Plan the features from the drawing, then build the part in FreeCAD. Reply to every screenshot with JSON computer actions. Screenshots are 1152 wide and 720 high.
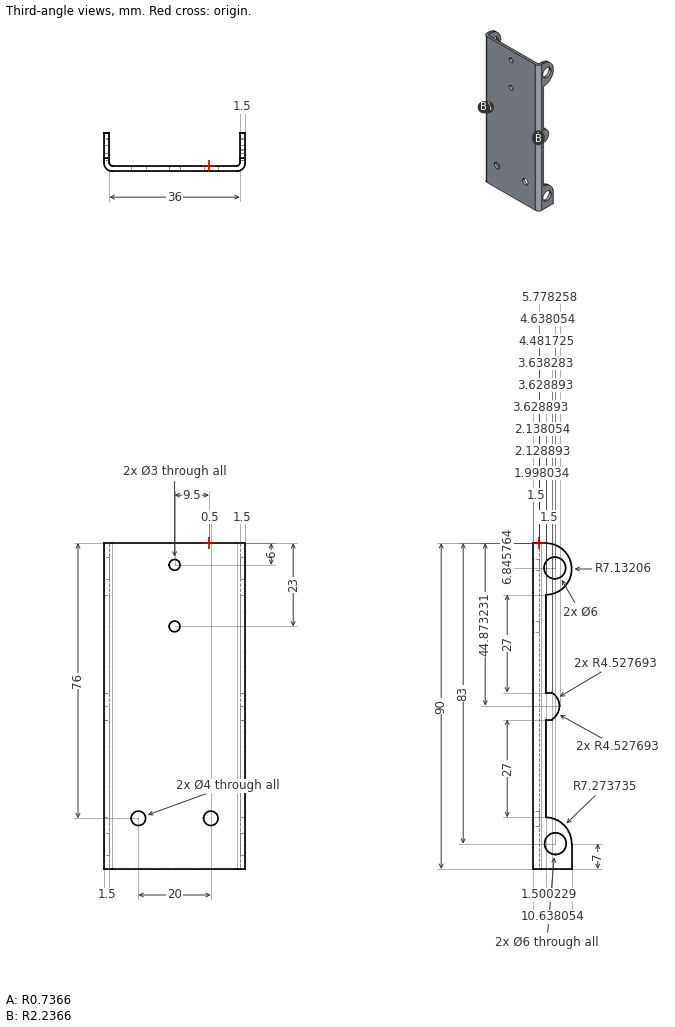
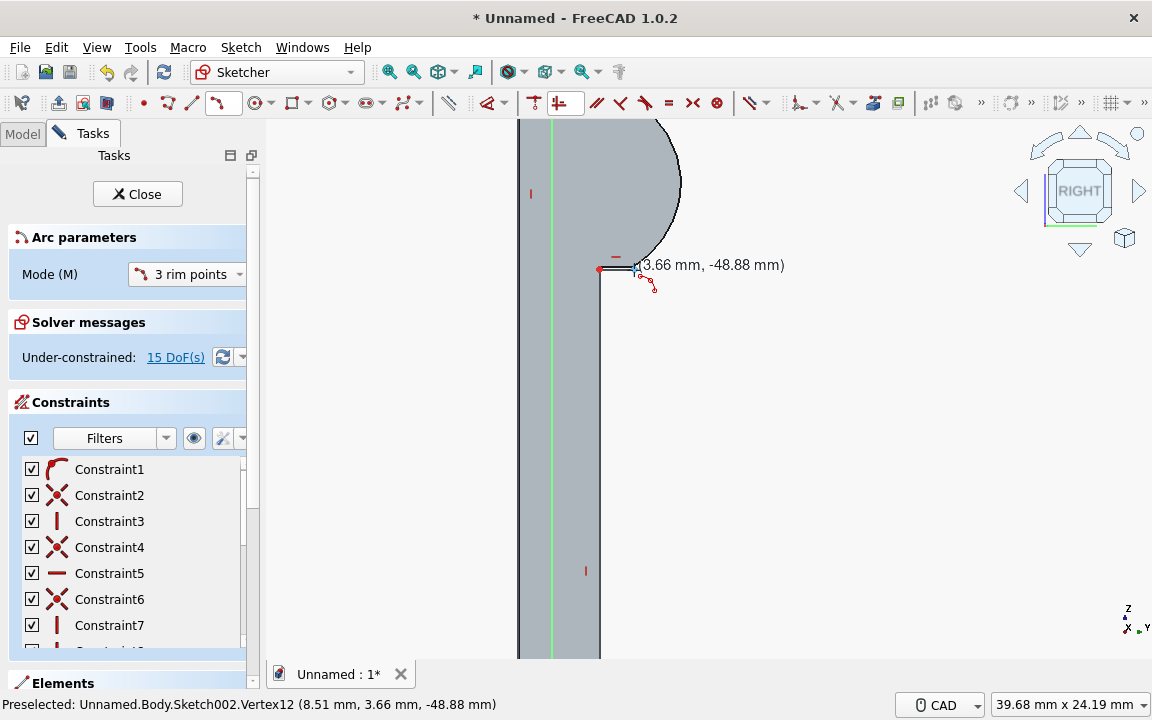
{"action": "scroll", "coordinate": [641, 430], "scroll_direction": "down", "scroll_amount": 9}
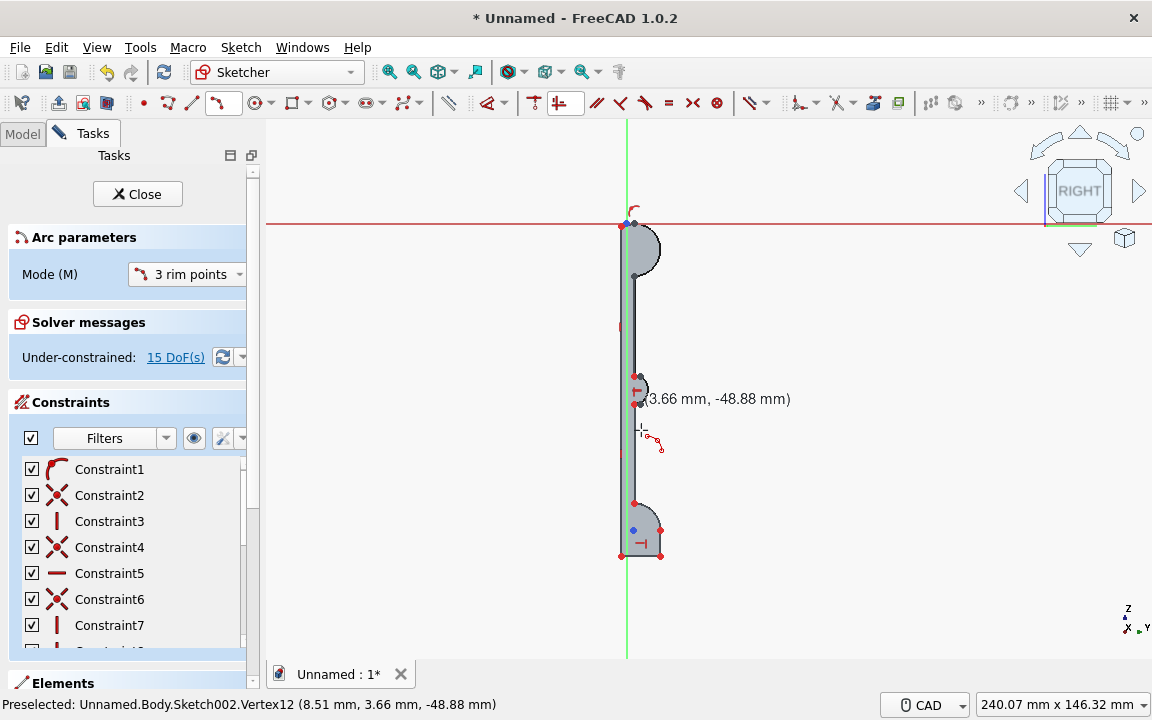
{"action": "left_click", "coordinate": [648, 389]}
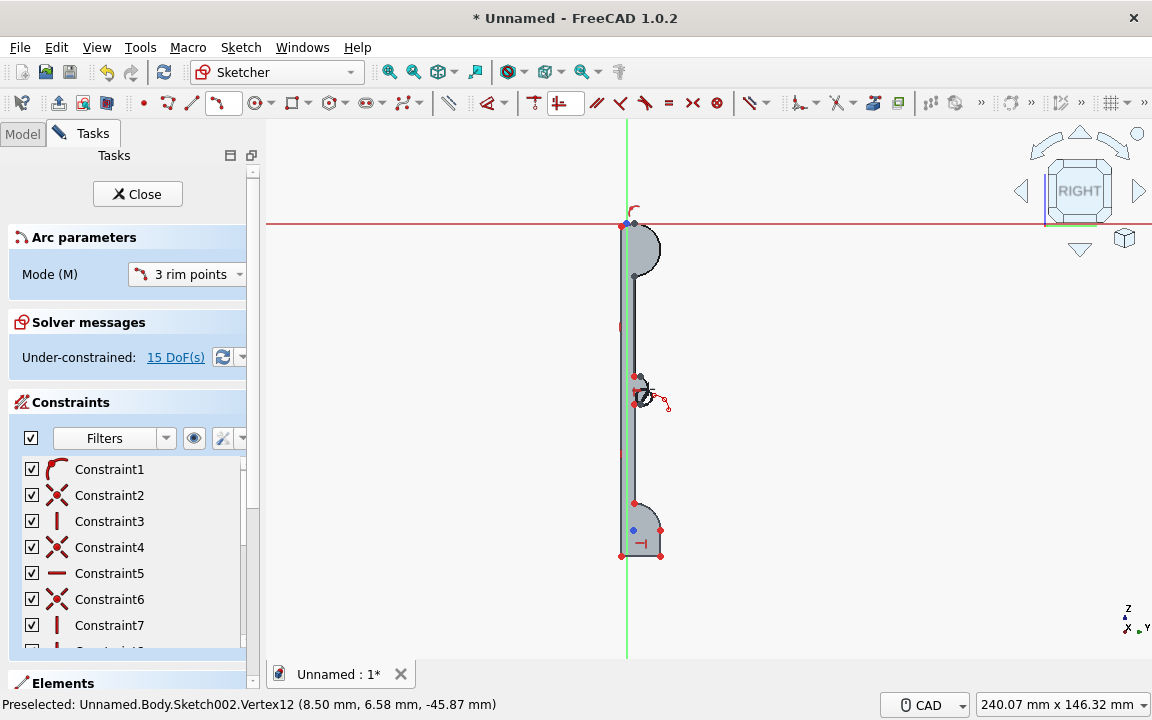
{"action": "scroll", "coordinate": [646, 397], "scroll_direction": "up", "scroll_amount": 11}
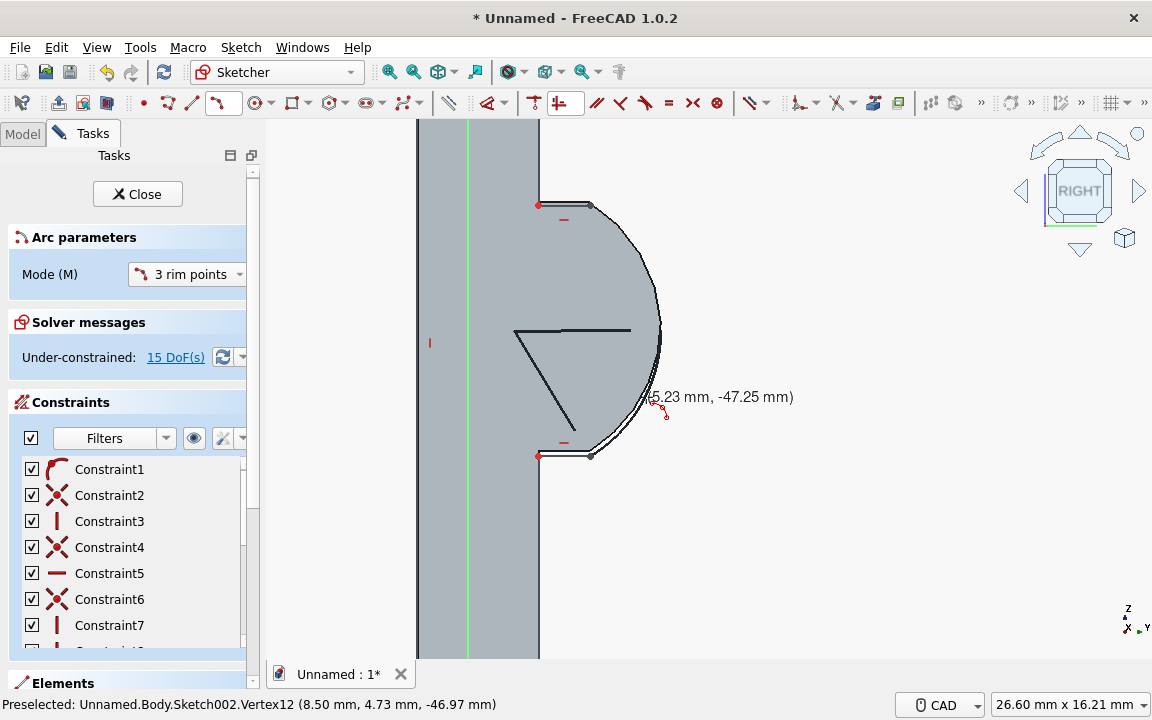
{"action": "left_click", "coordinate": [642, 396]}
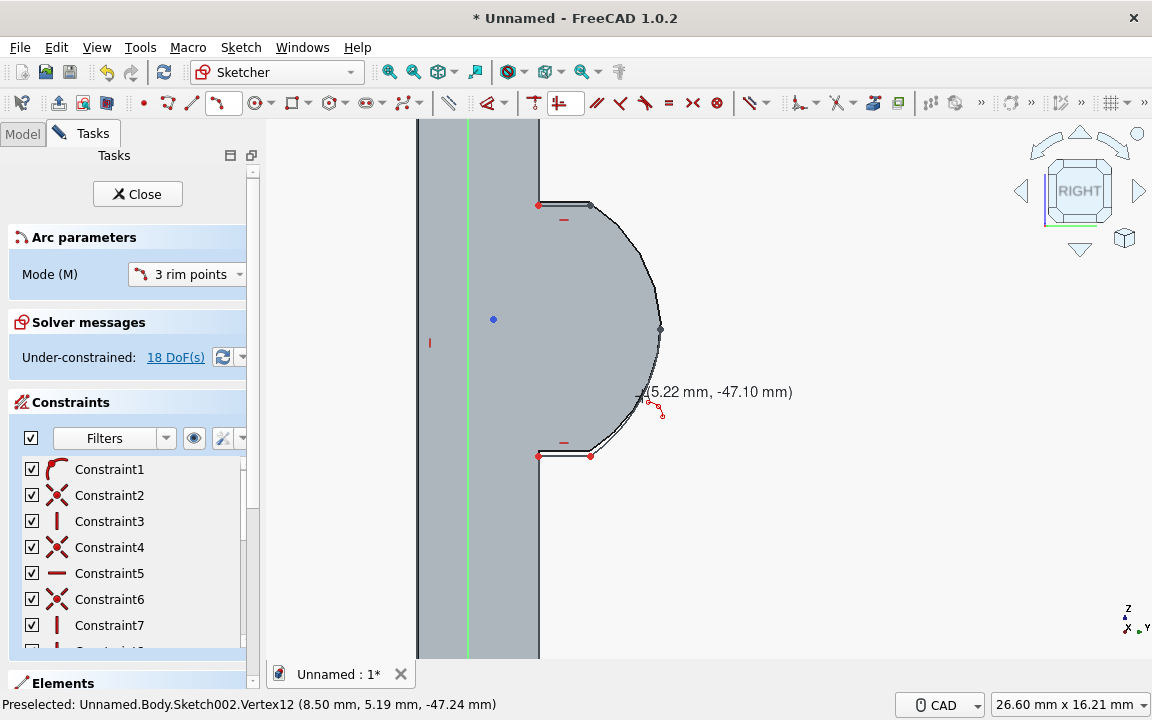
{"action": "scroll", "coordinate": [646, 397], "scroll_direction": "down", "scroll_amount": 11}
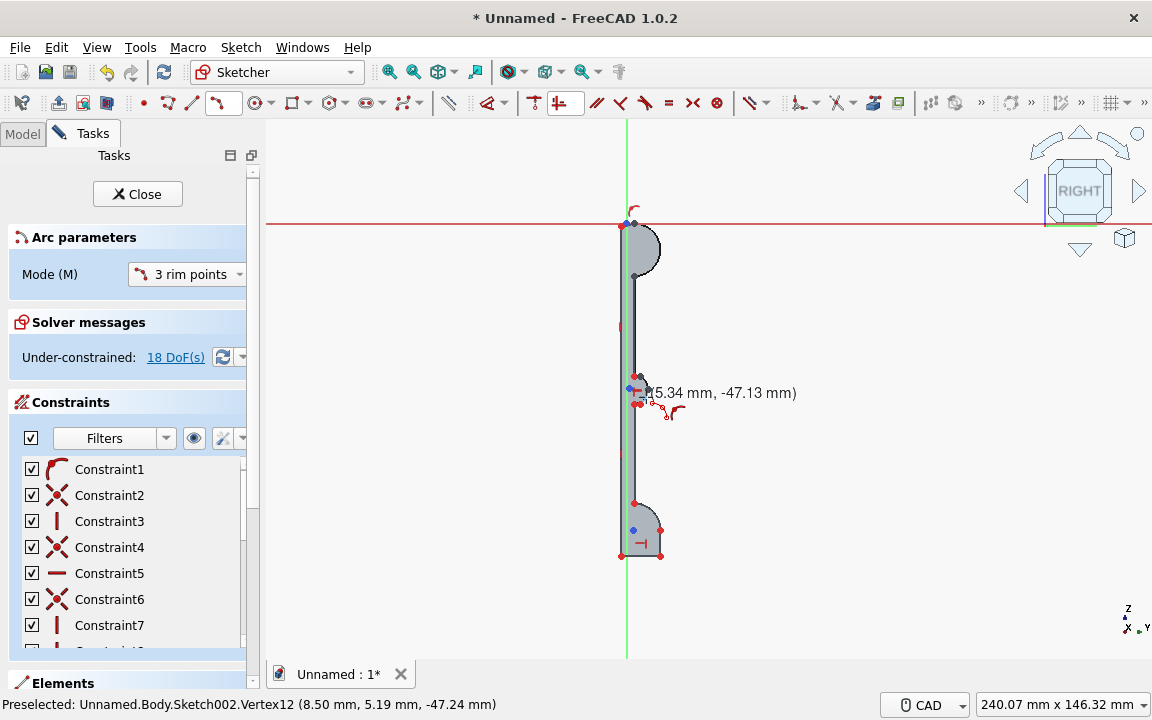
{"action": "left_click", "coordinate": [648, 390]}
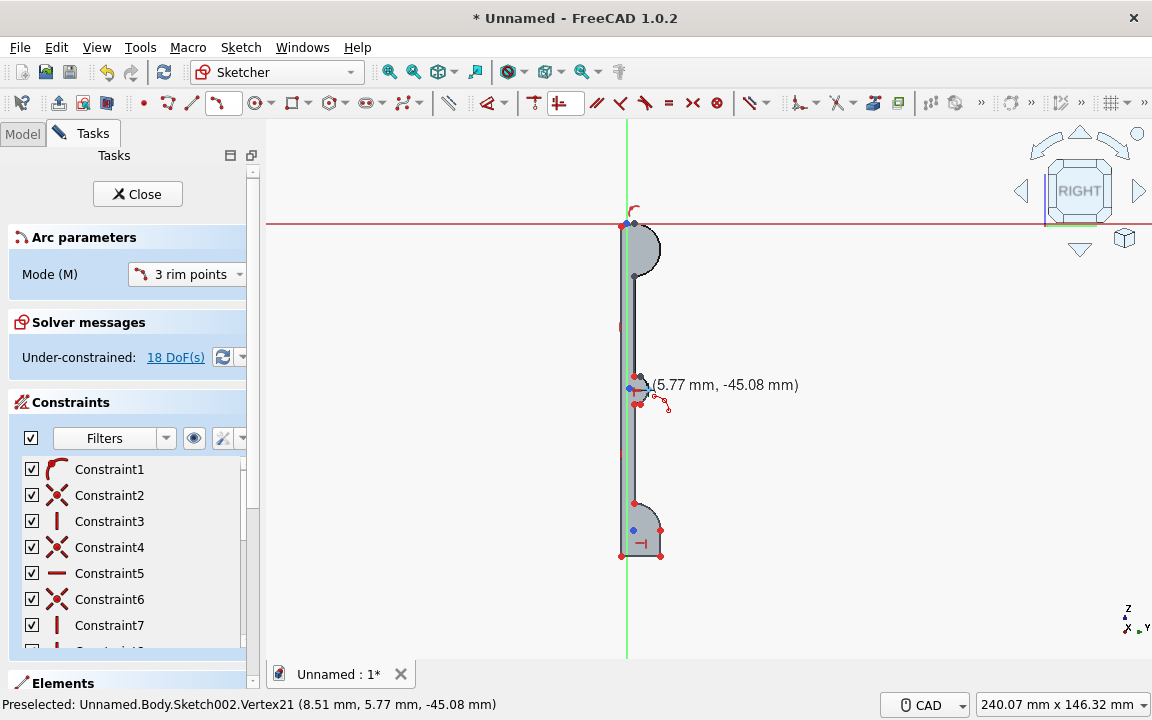
{"action": "scroll", "coordinate": [640, 376], "scroll_direction": "up", "scroll_amount": 9}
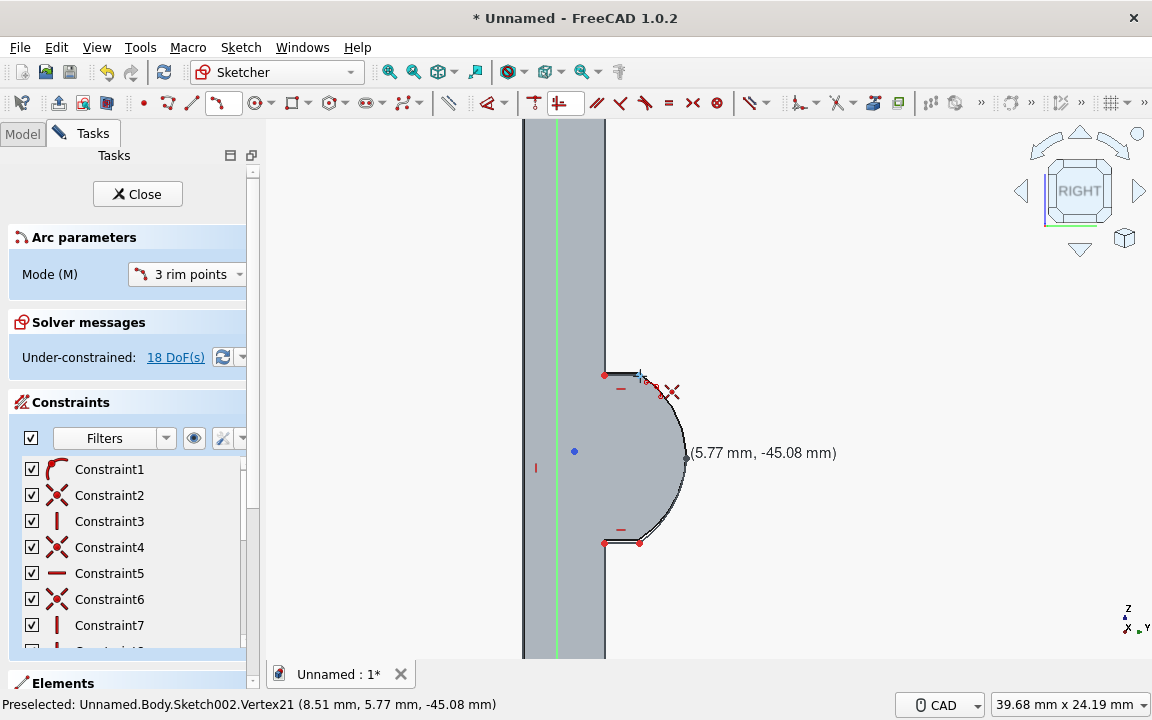
{"action": "left_click", "coordinate": [639, 375]}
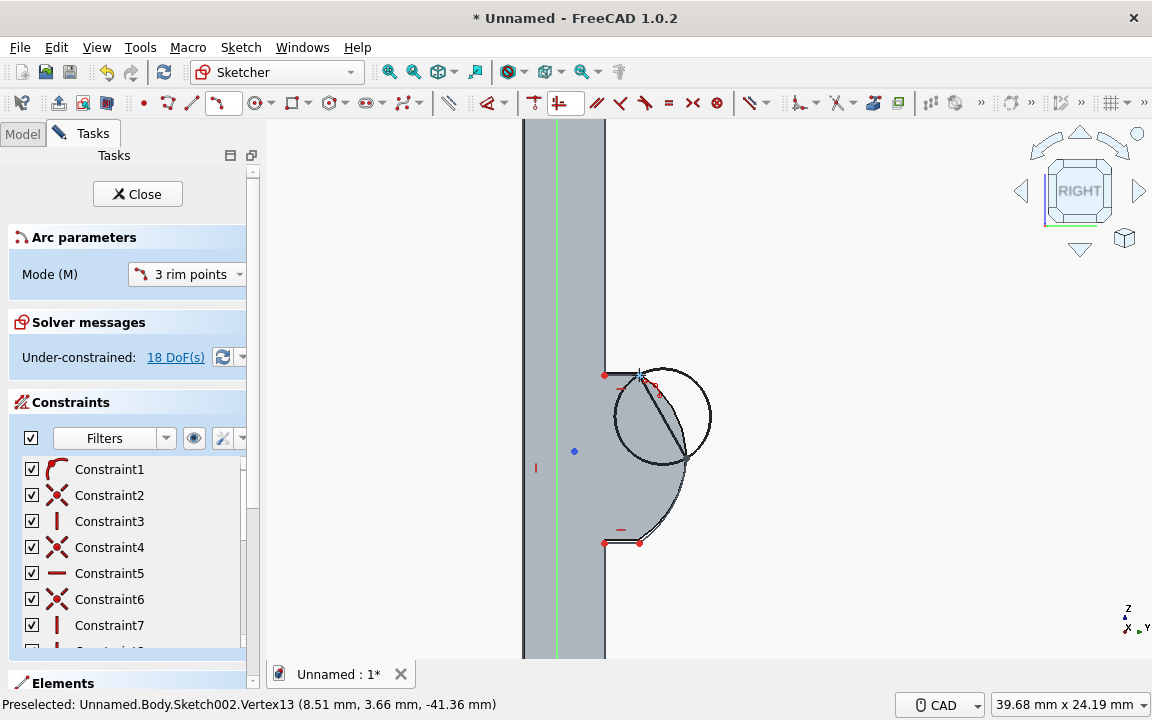
{"action": "scroll", "coordinate": [672, 407], "scroll_direction": "up", "scroll_amount": 2}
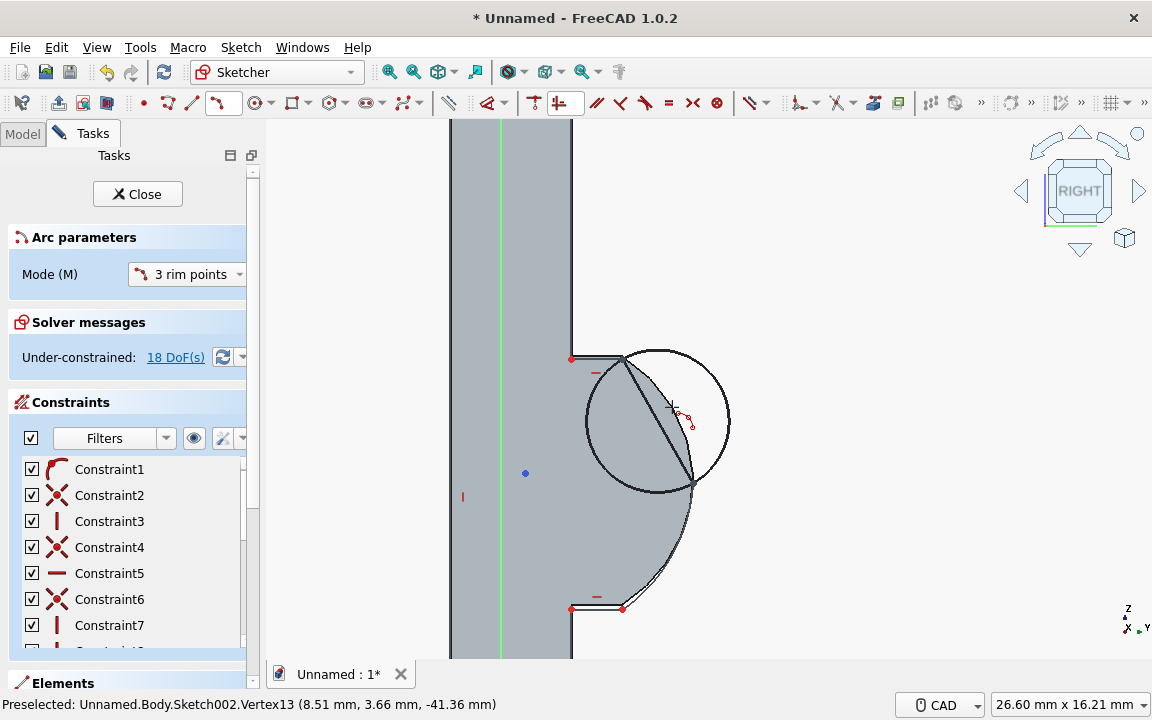
{"action": "left_click", "coordinate": [672, 407]}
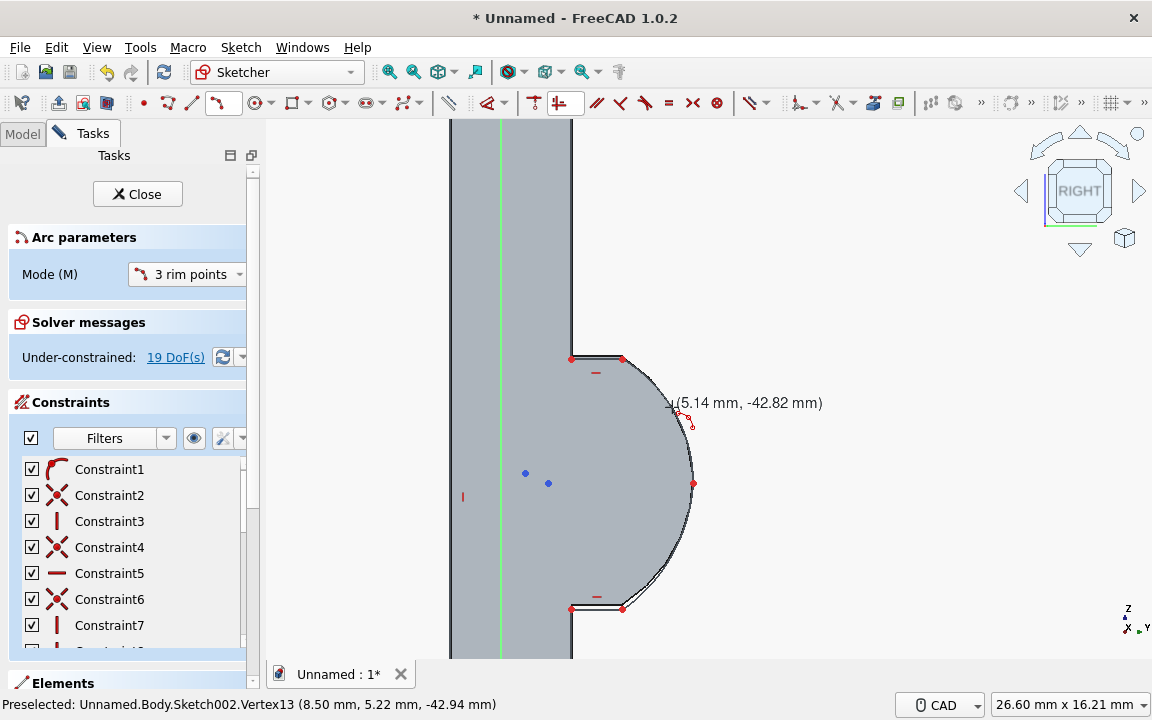
{"action": "scroll", "coordinate": [642, 378], "scroll_direction": "down", "scroll_amount": 11}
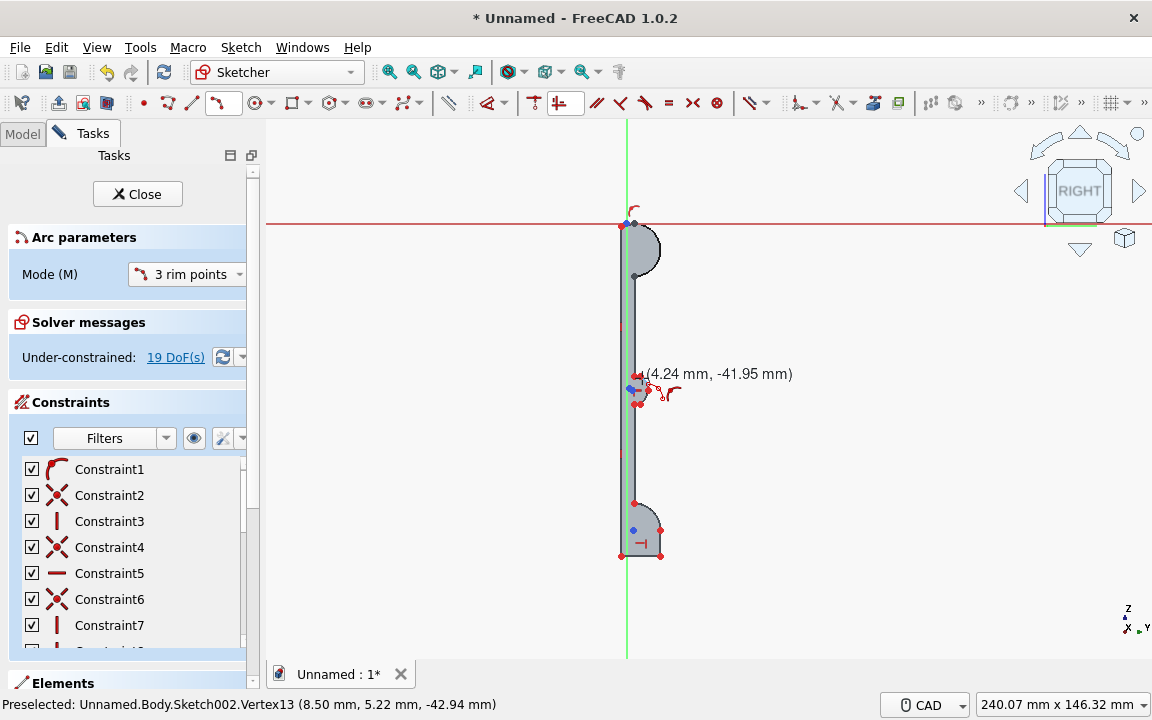
{"action": "scroll", "coordinate": [635, 276], "scroll_direction": "up", "scroll_amount": 4}